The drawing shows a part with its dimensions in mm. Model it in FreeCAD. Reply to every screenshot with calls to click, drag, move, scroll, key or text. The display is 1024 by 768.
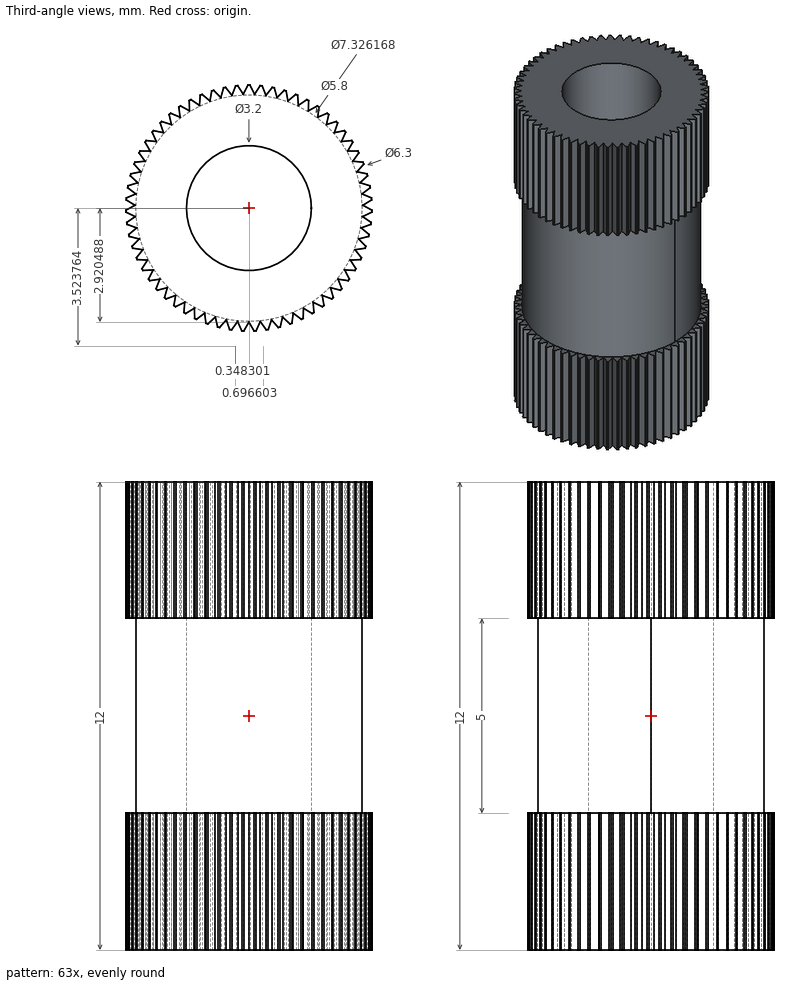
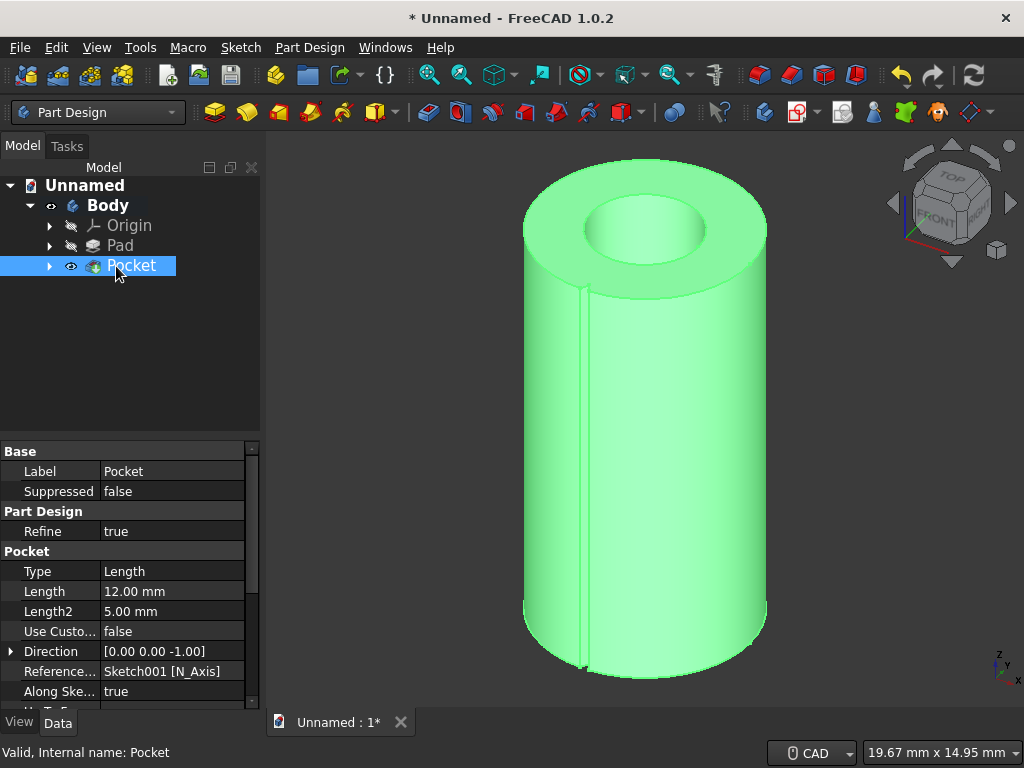
click(90, 76)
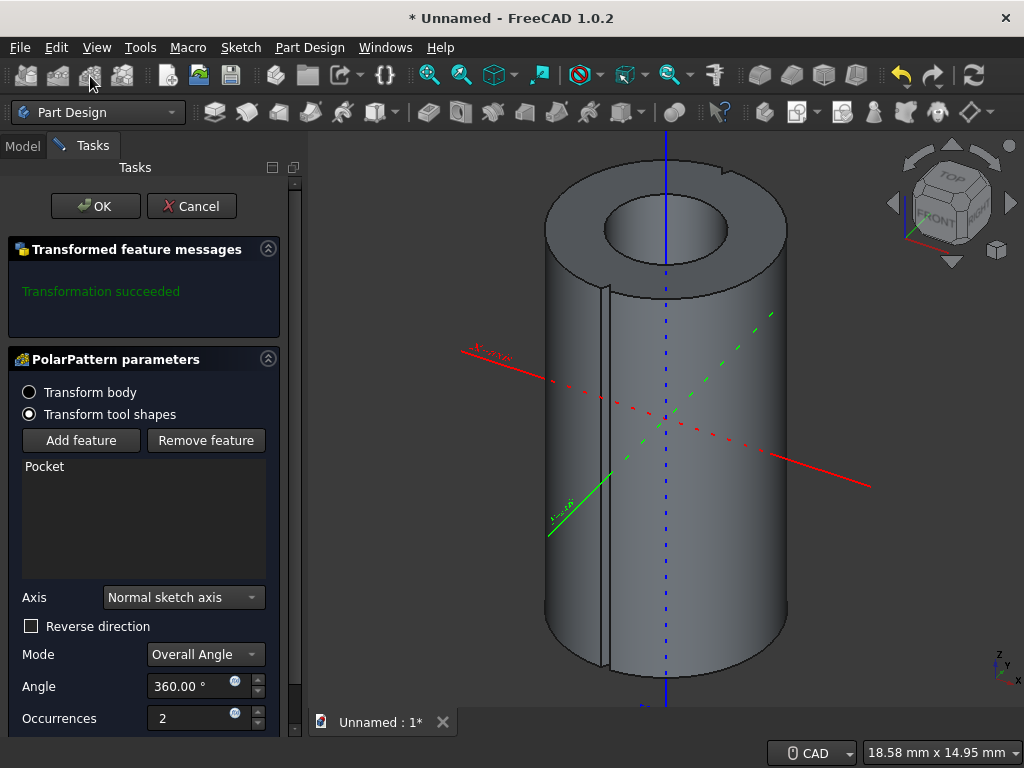
click(184, 598)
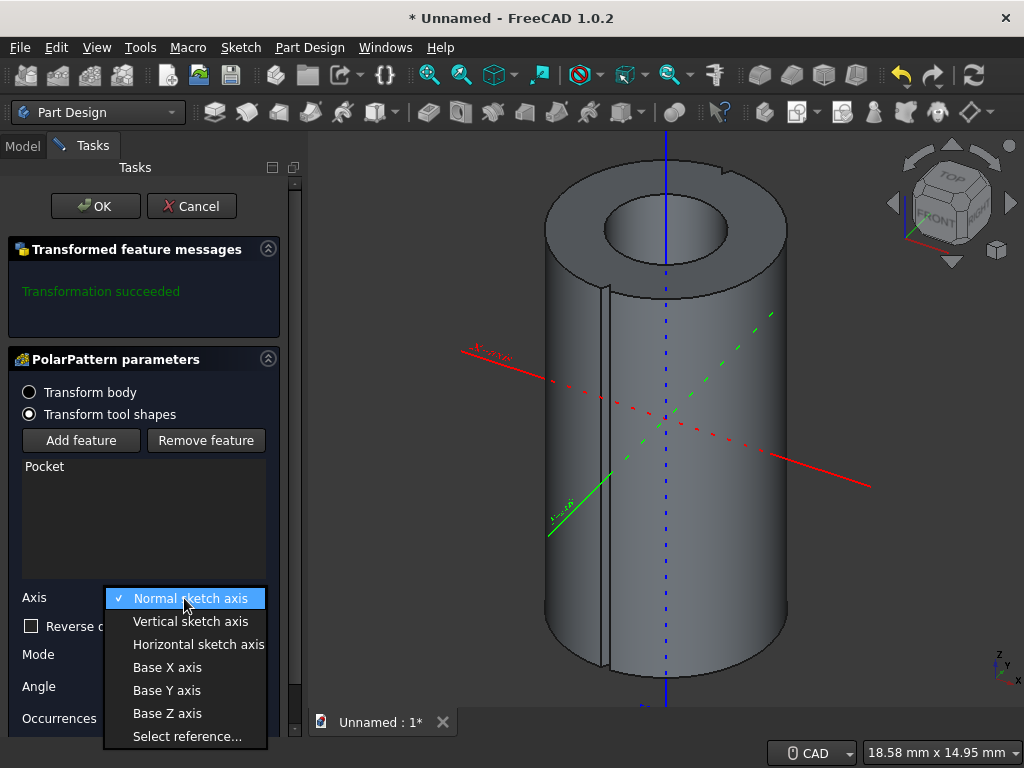
click(184, 714)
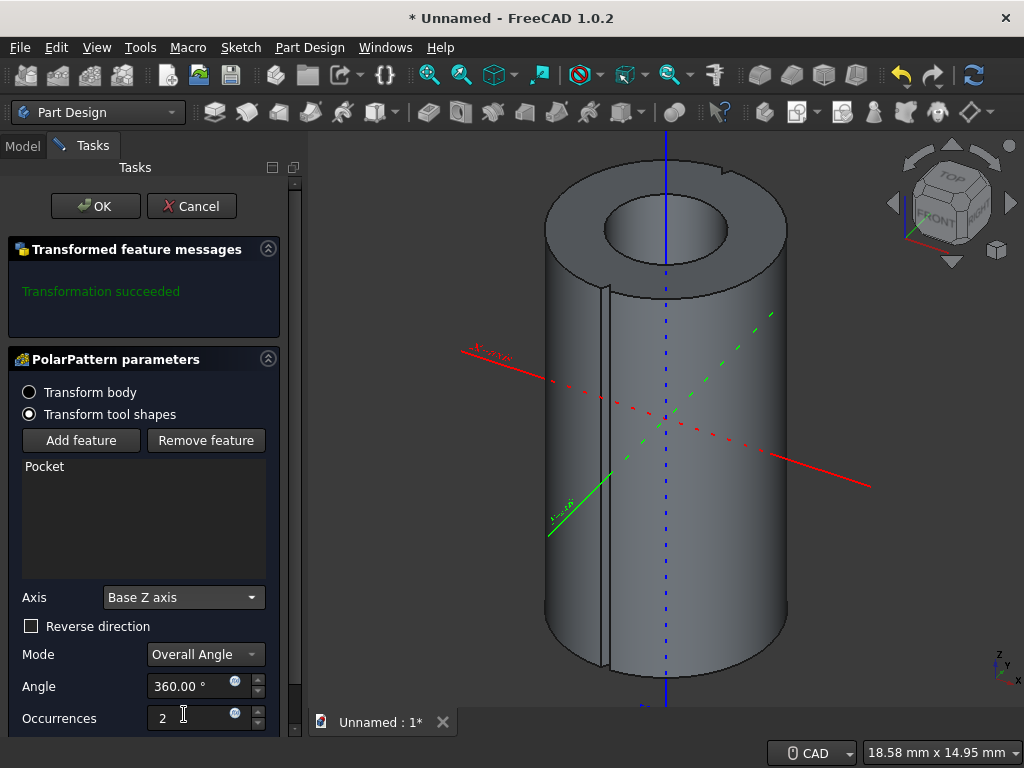
triple_click(198, 718)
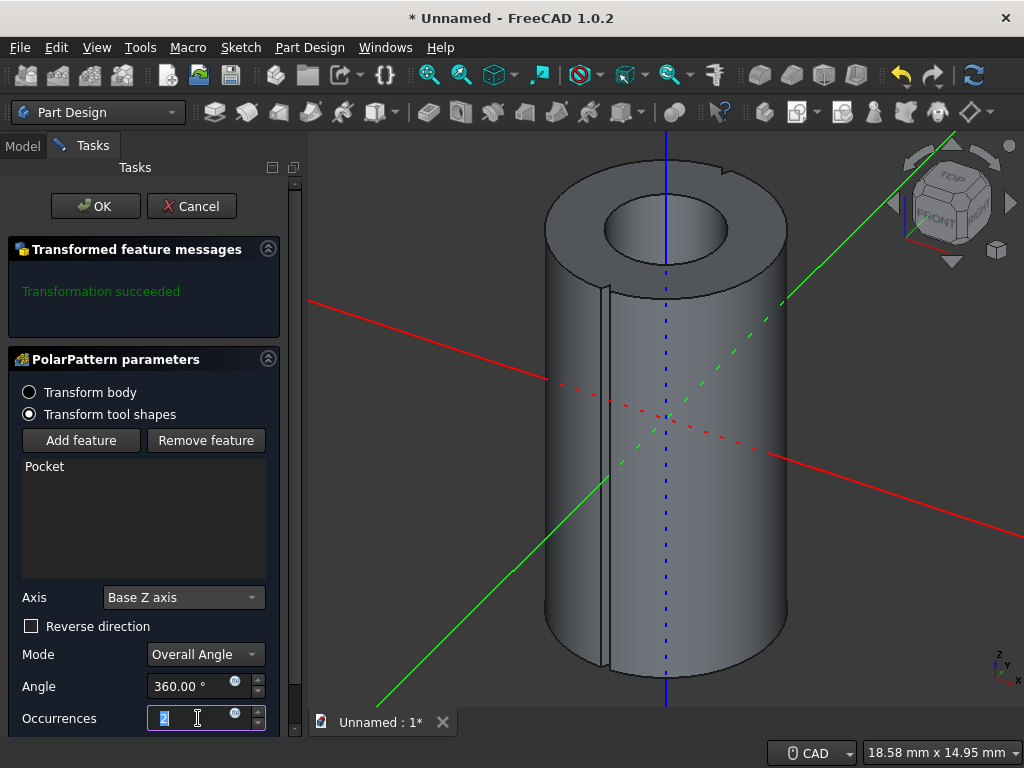
text(63)
key(Tab)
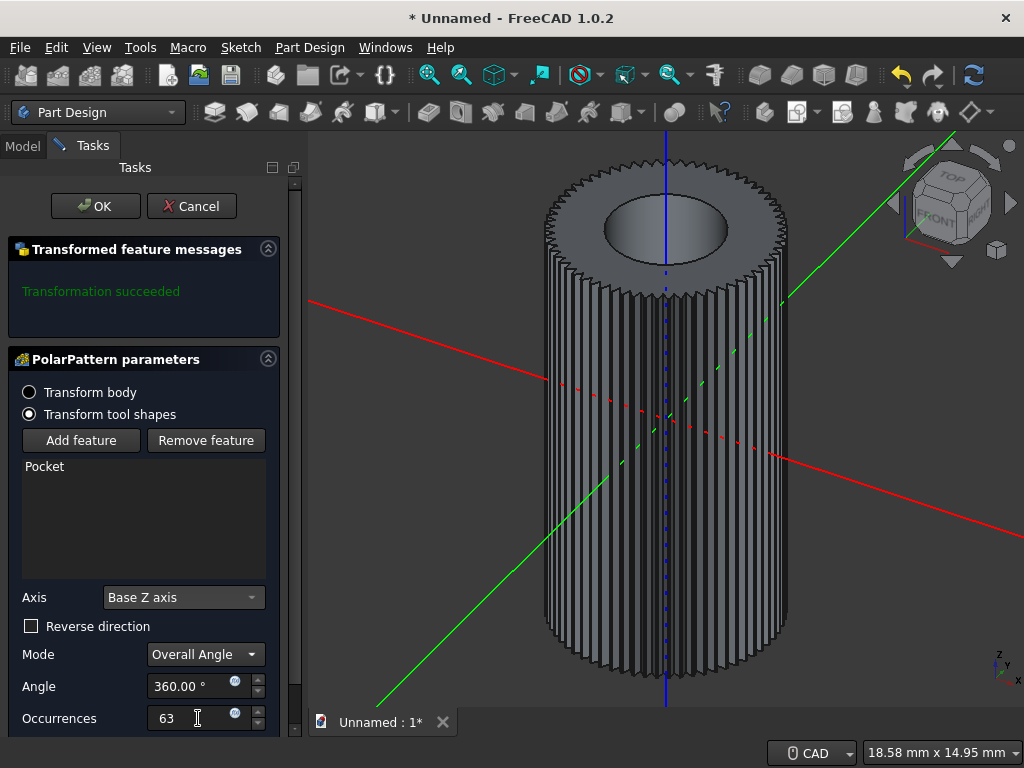
click(96, 206)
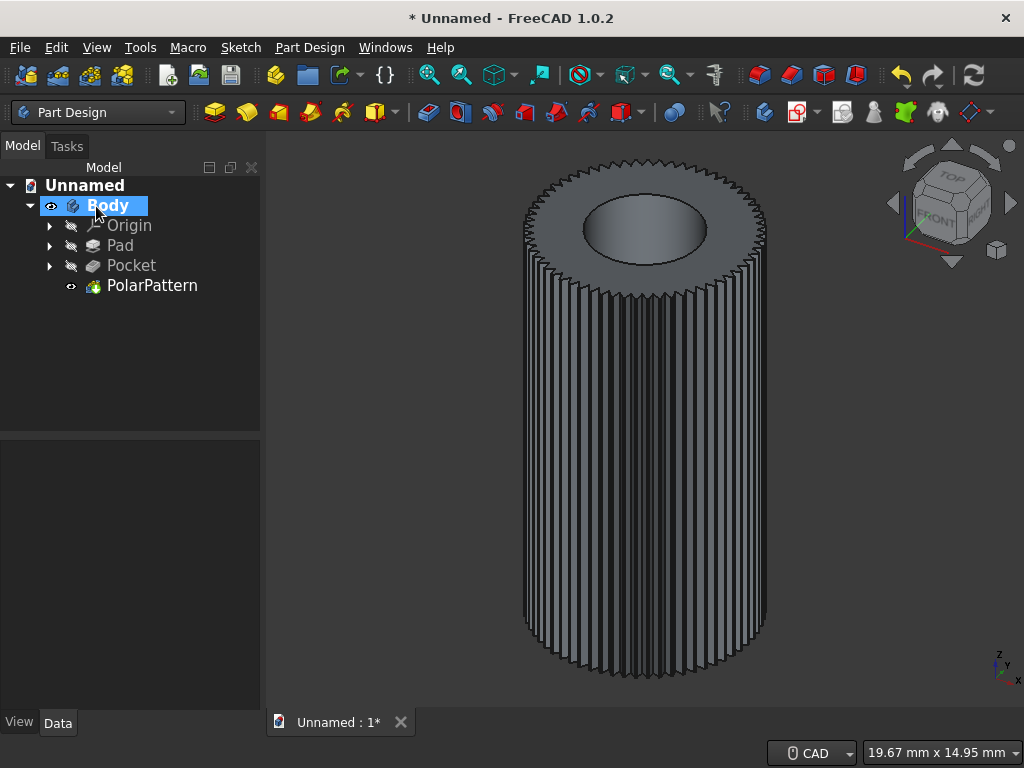
click(798, 112)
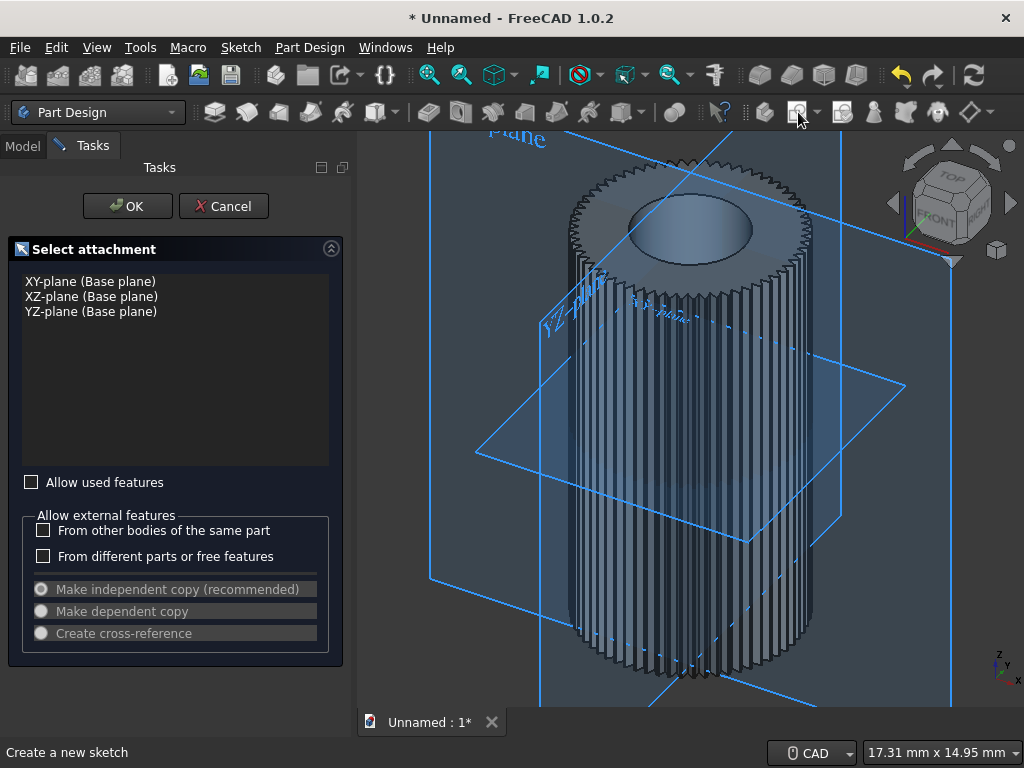
click(82, 282)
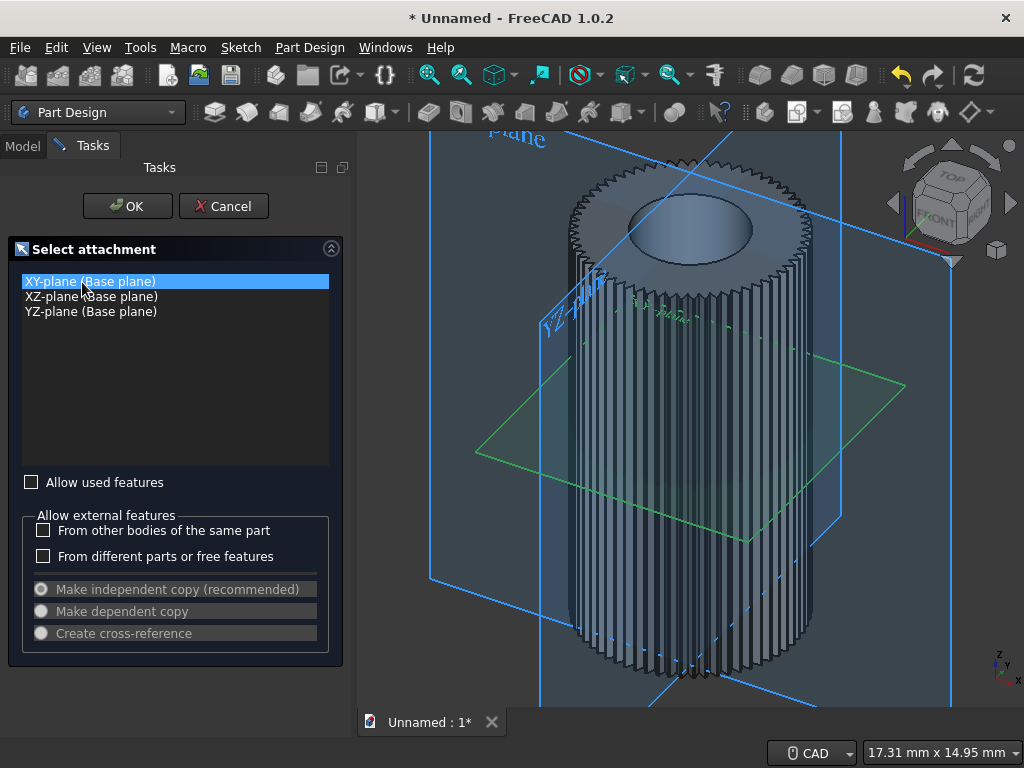
click(128, 206)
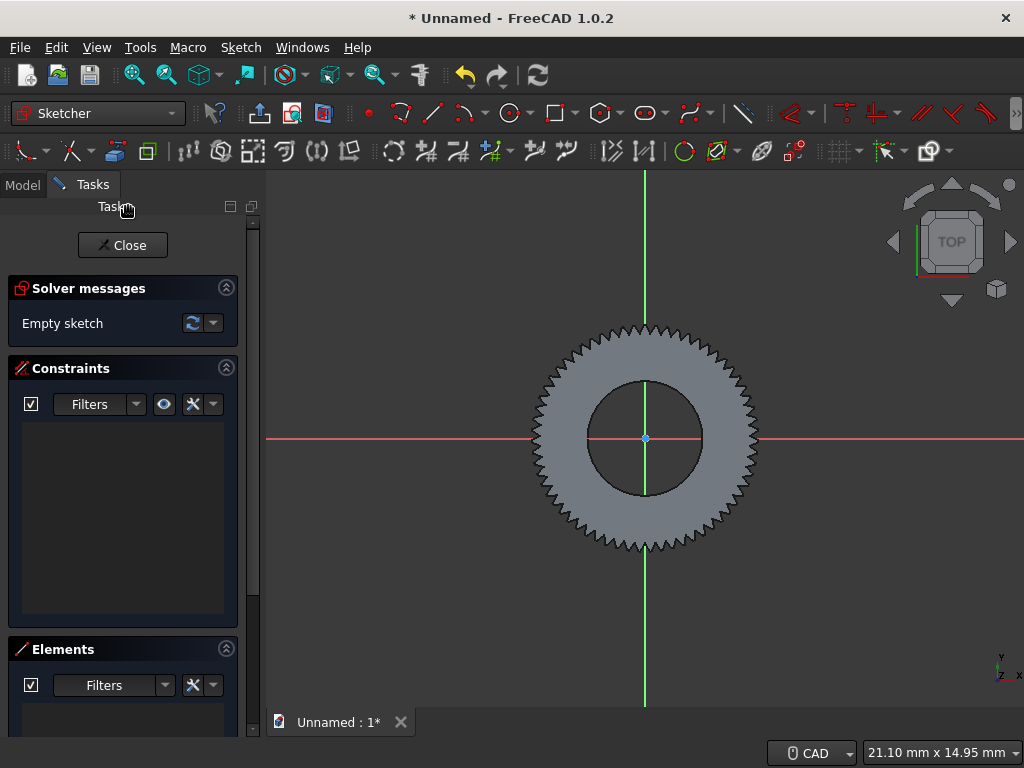
click(324, 114)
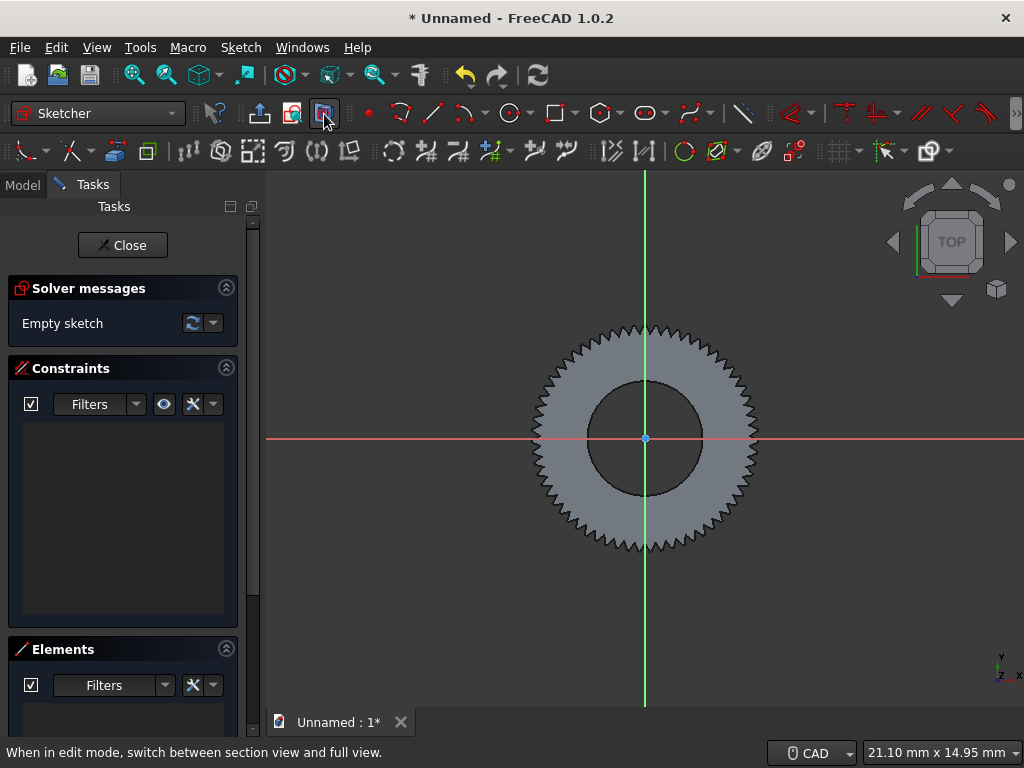
click(510, 114)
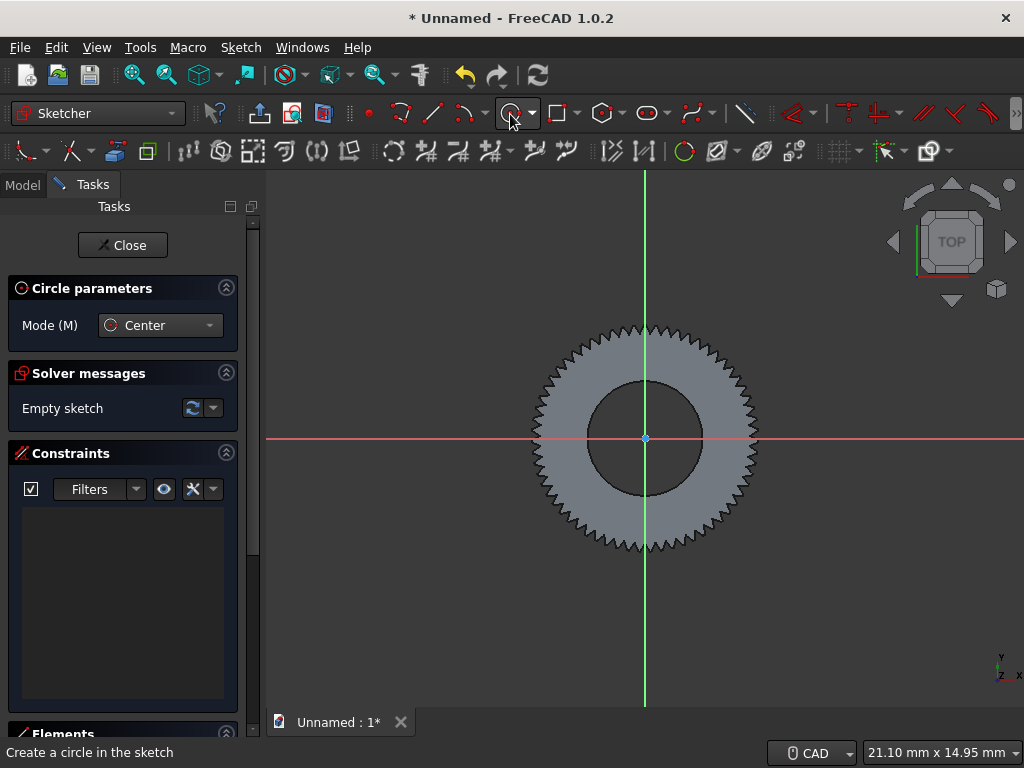
click(645, 438)
click(738, 345)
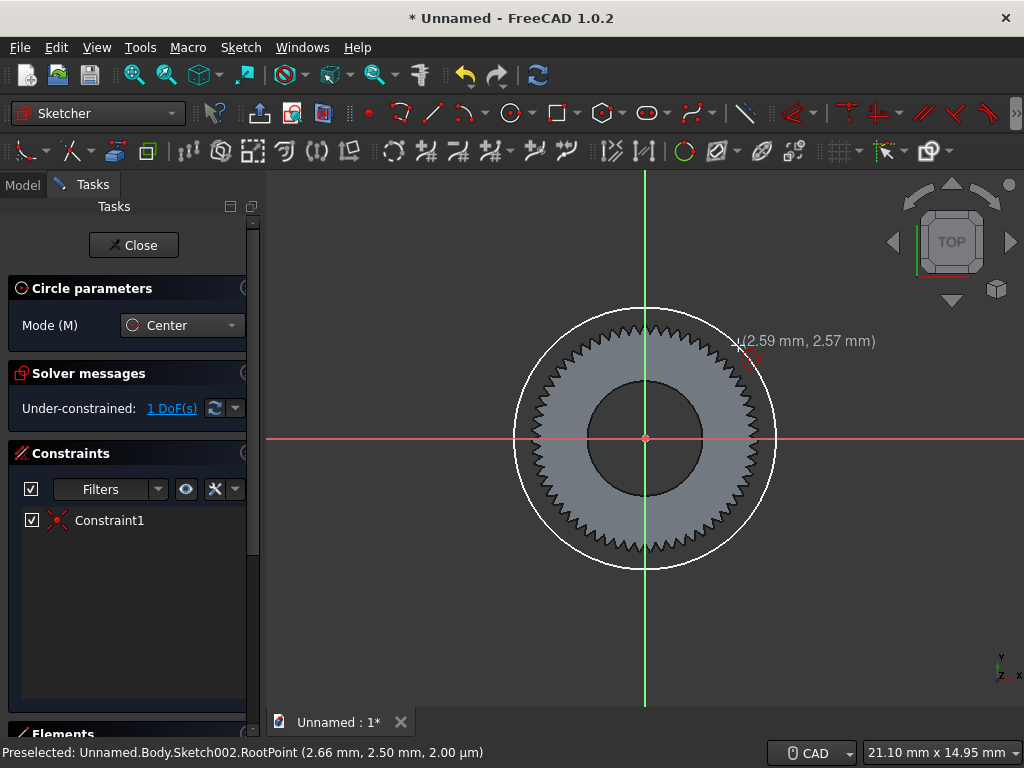
click(645, 438)
click(719, 365)
key(Escape)